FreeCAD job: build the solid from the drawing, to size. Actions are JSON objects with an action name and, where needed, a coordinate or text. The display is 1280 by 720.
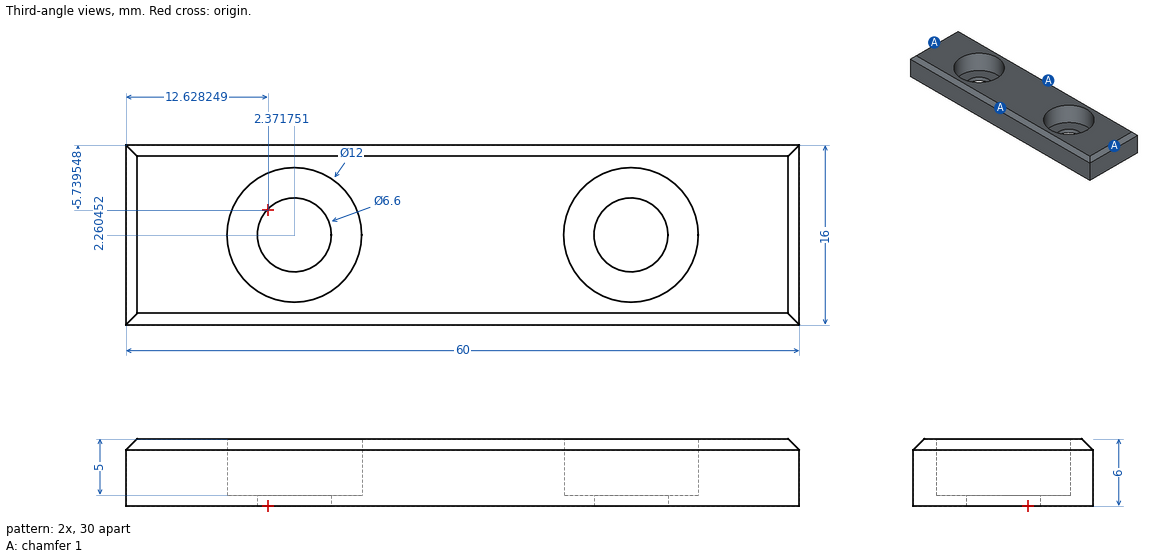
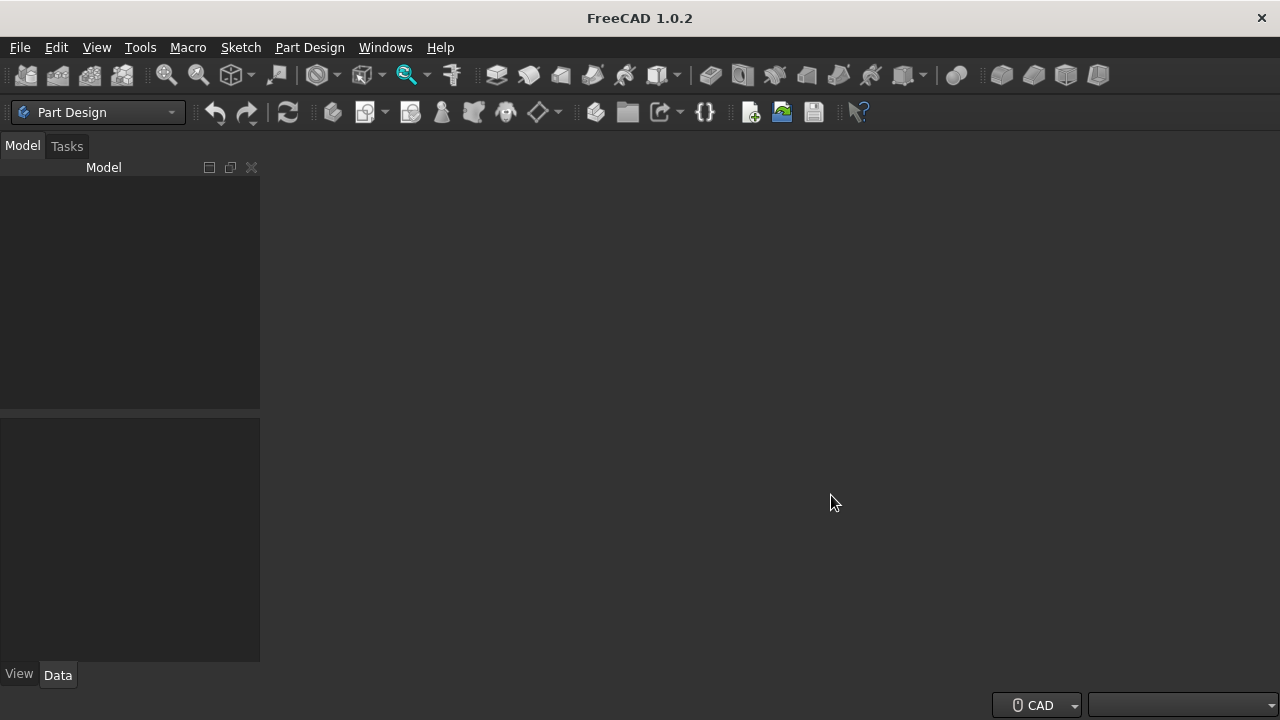
{"action": "left_click", "coordinate": [750, 112]}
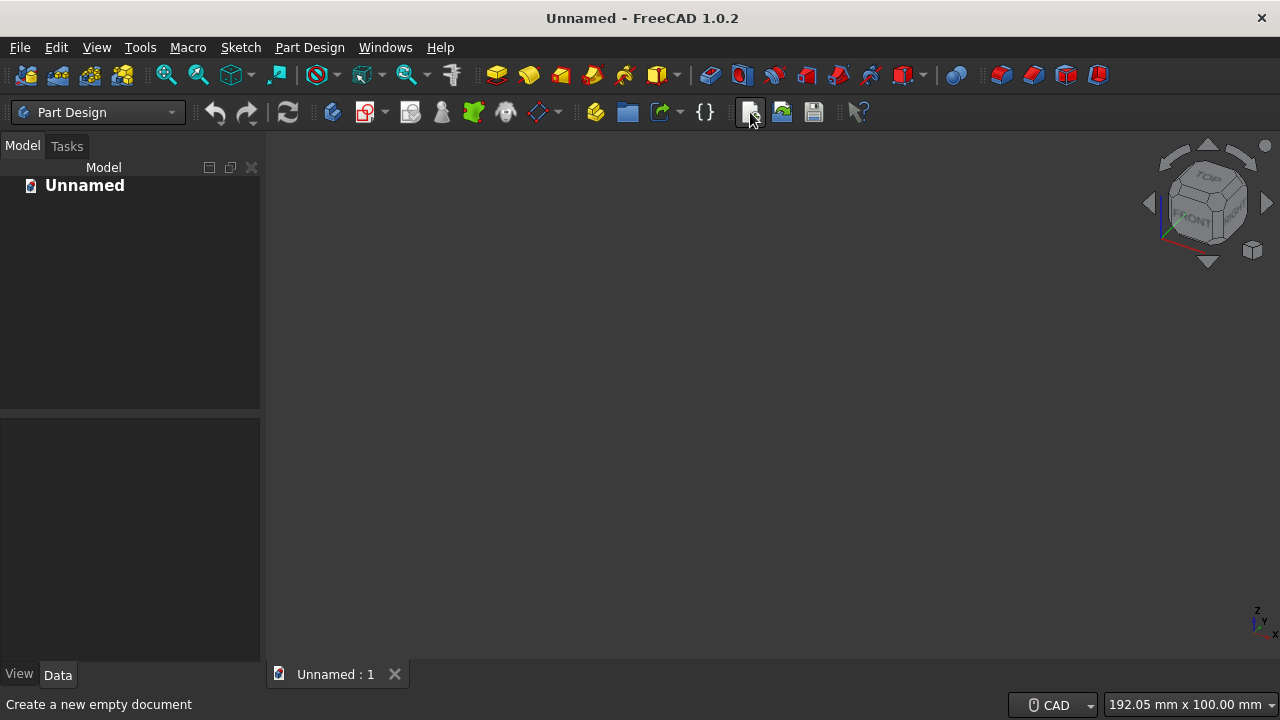
{"action": "left_click", "coordinate": [366, 112]}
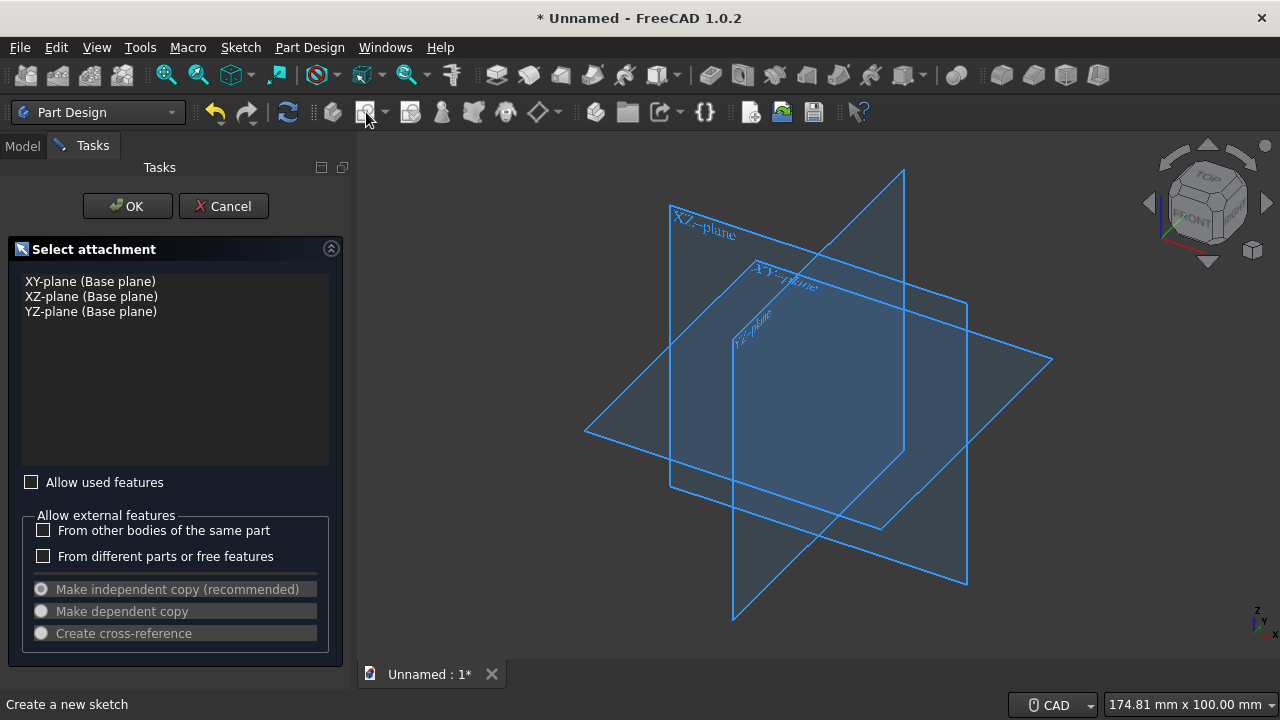
{"action": "left_click", "coordinate": [82, 282]}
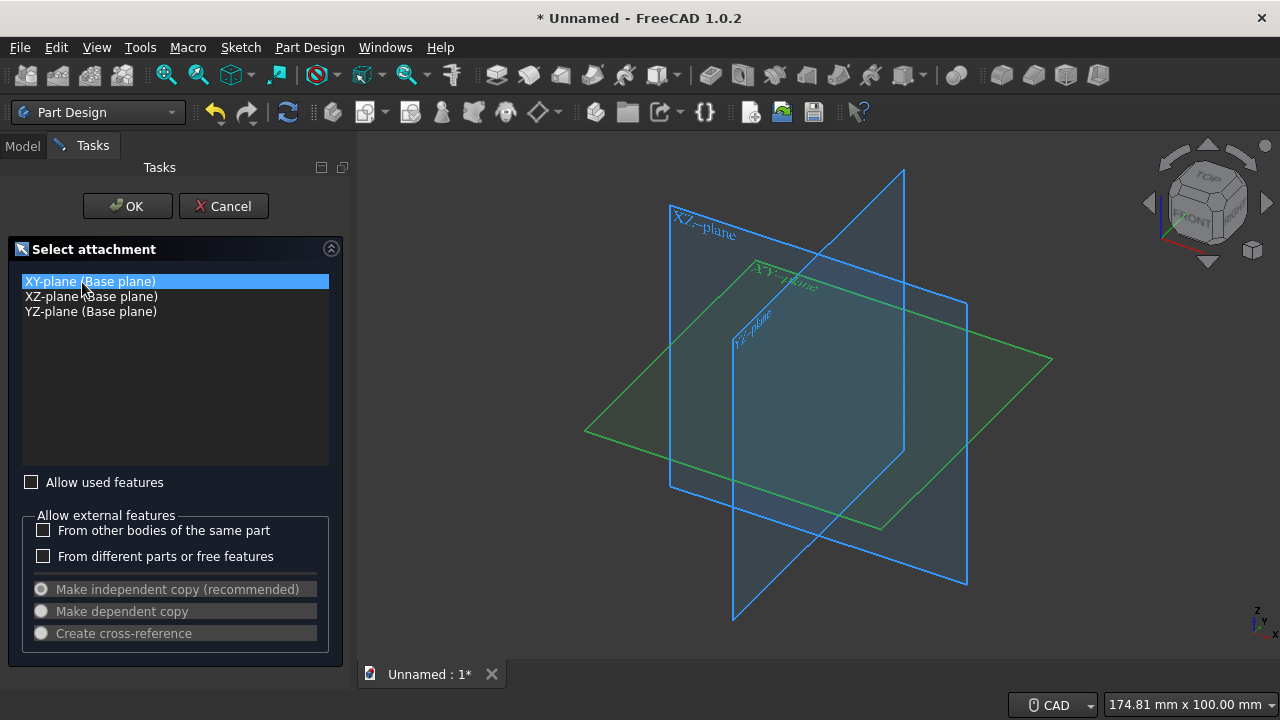
{"action": "left_click", "coordinate": [128, 206]}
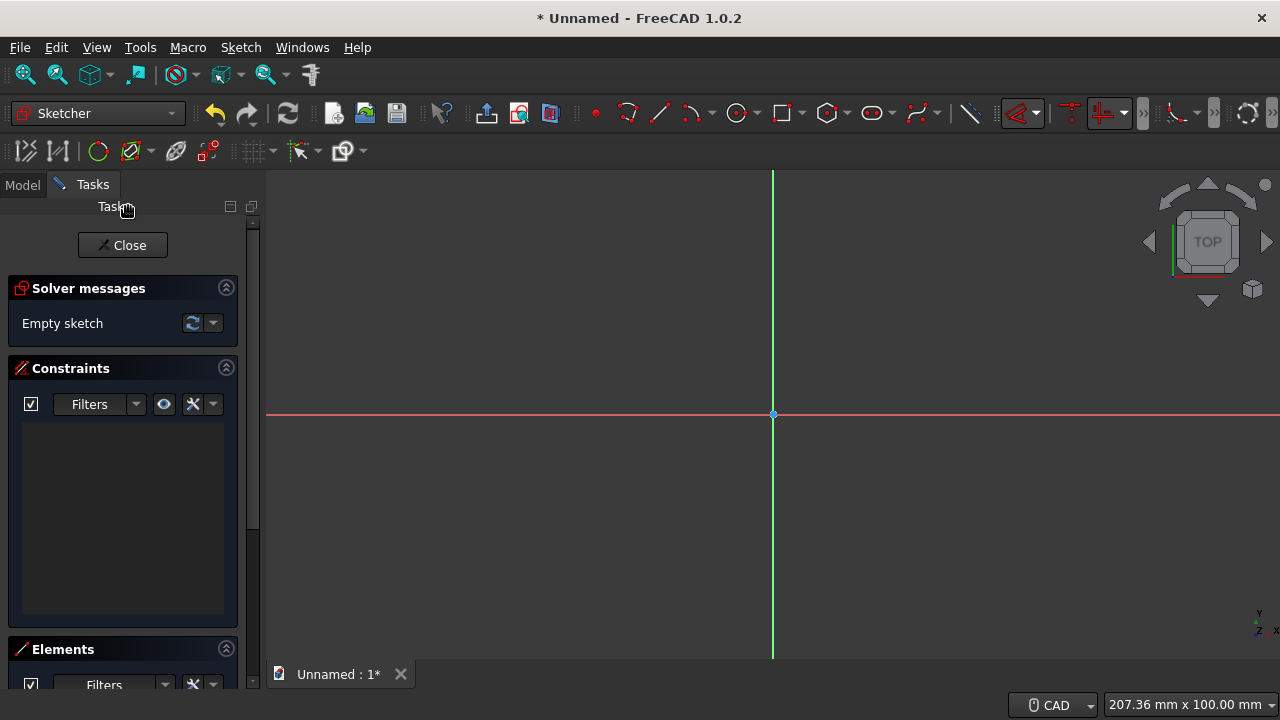
{"action": "scroll", "coordinate": [1045, 439], "scroll_direction": "up", "scroll_amount": 3}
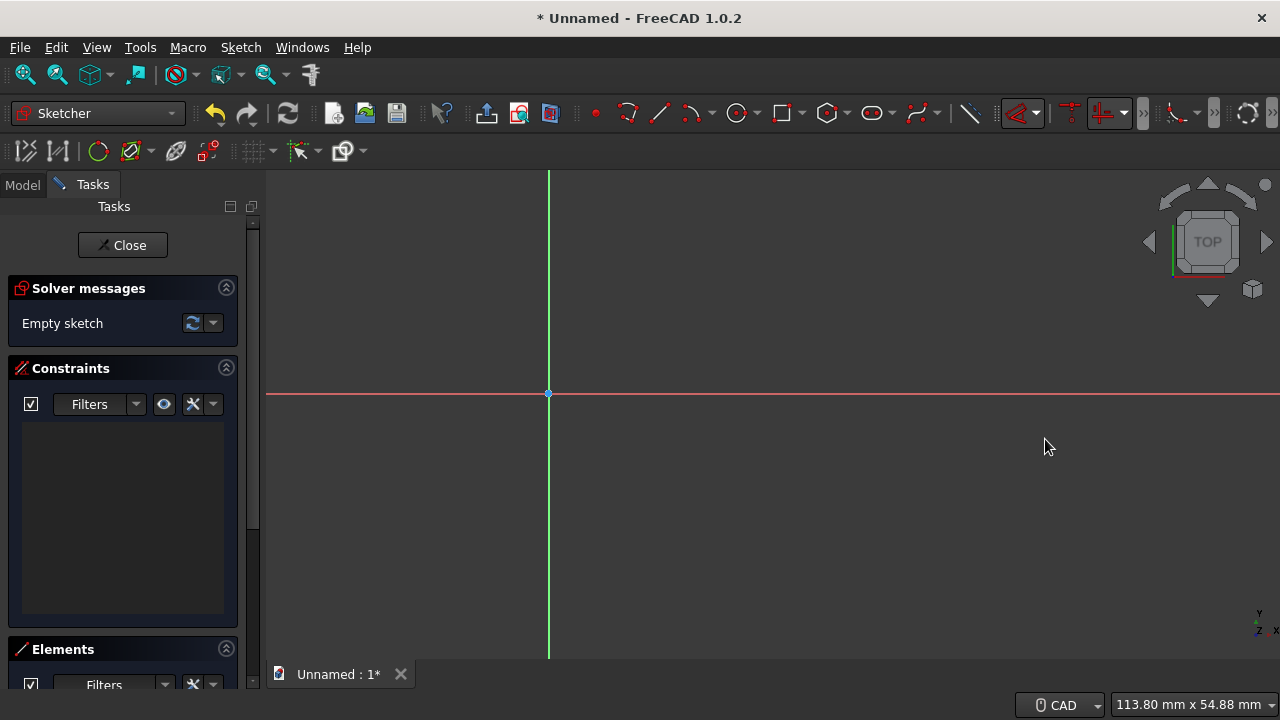
{"action": "left_click", "coordinate": [782, 114]}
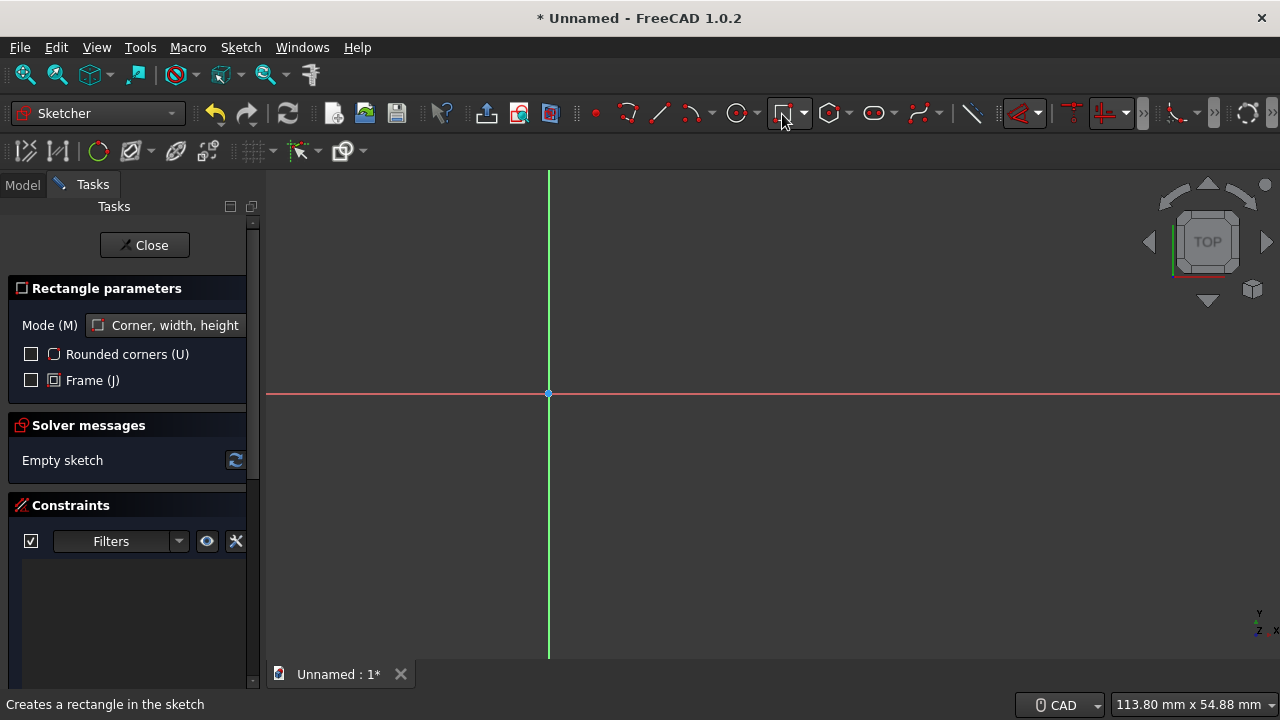
{"action": "left_click", "coordinate": [436, 343]}
{"action": "mouse_move", "coordinate": [971, 485]}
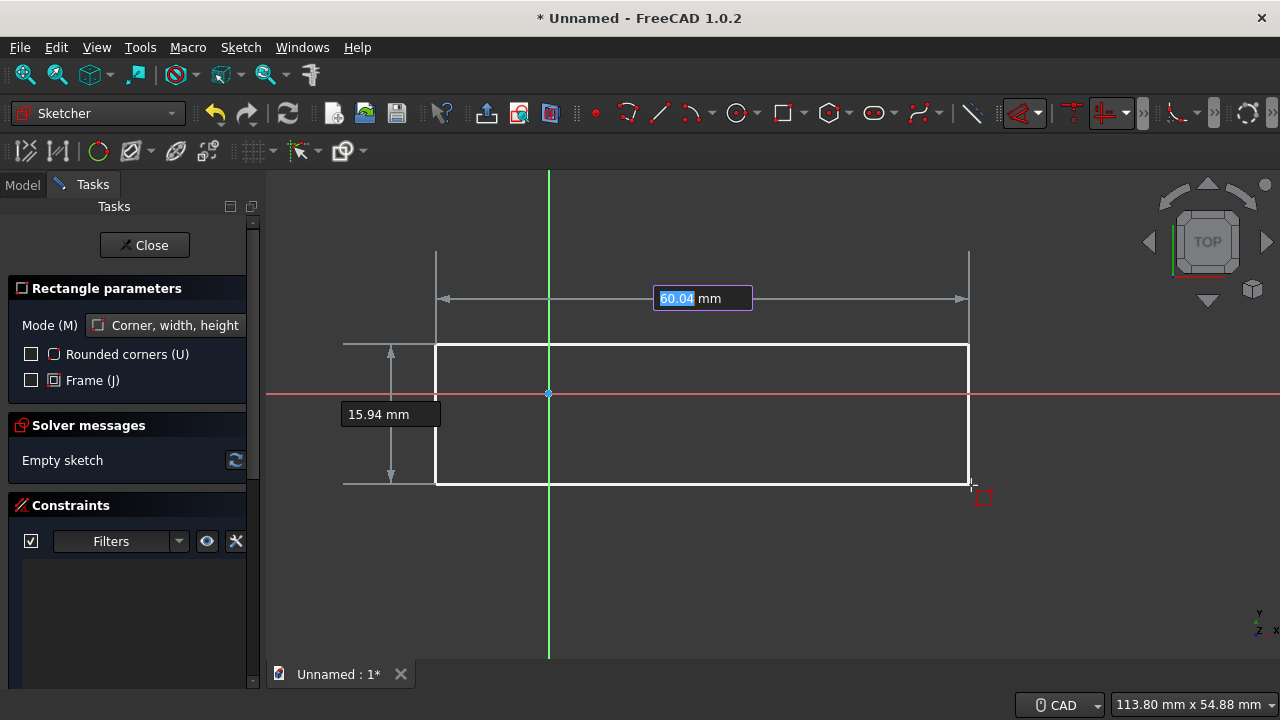
{"action": "type", "text": "60"}
{"action": "key", "text": "Tab"}
{"action": "type", "text": "16"}
{"action": "key", "text": "Return"}
{"action": "key", "text": "Escape"}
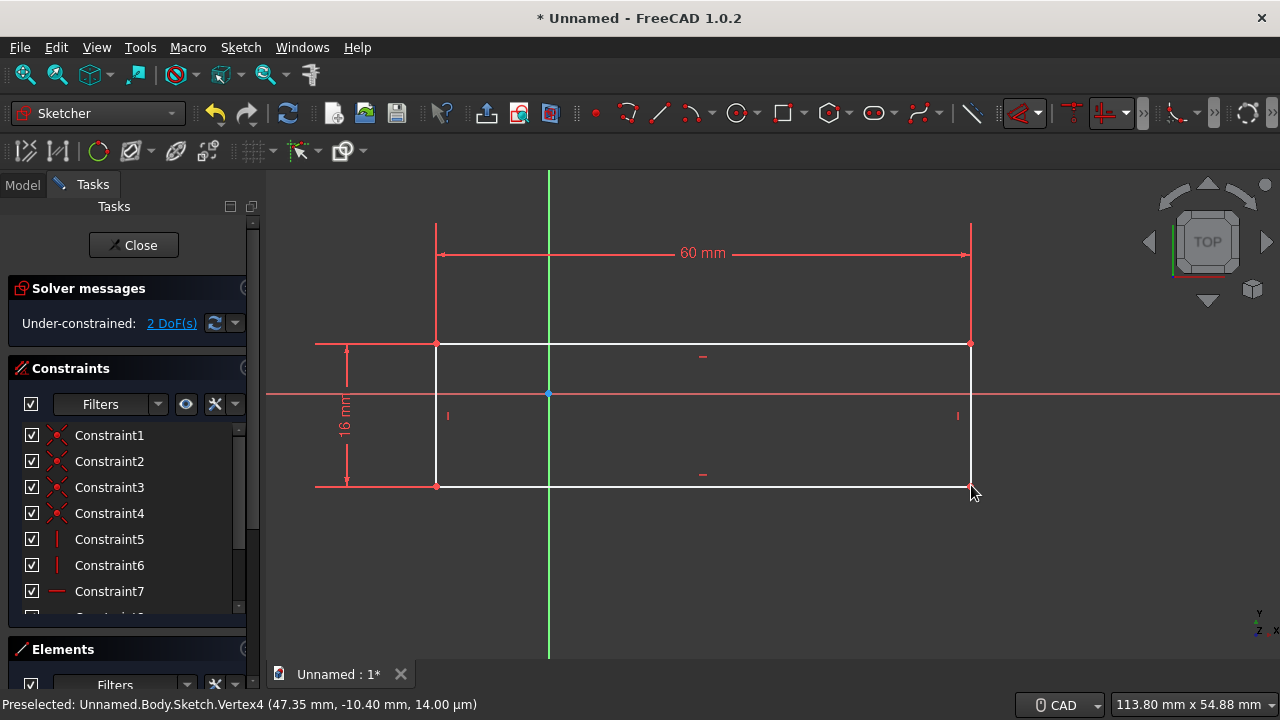
{"action": "left_click", "coordinate": [1018, 114]}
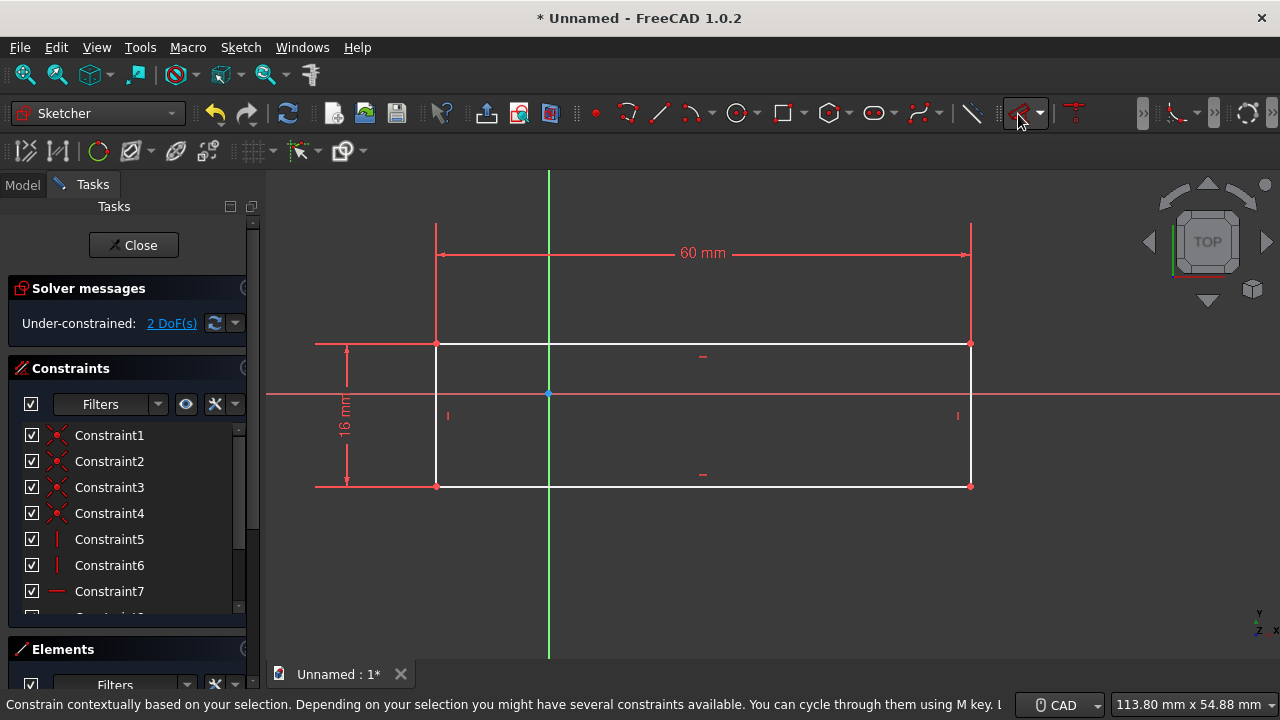
{"action": "left_click", "coordinate": [436, 344]}
{"action": "left_click", "coordinate": [402, 369]}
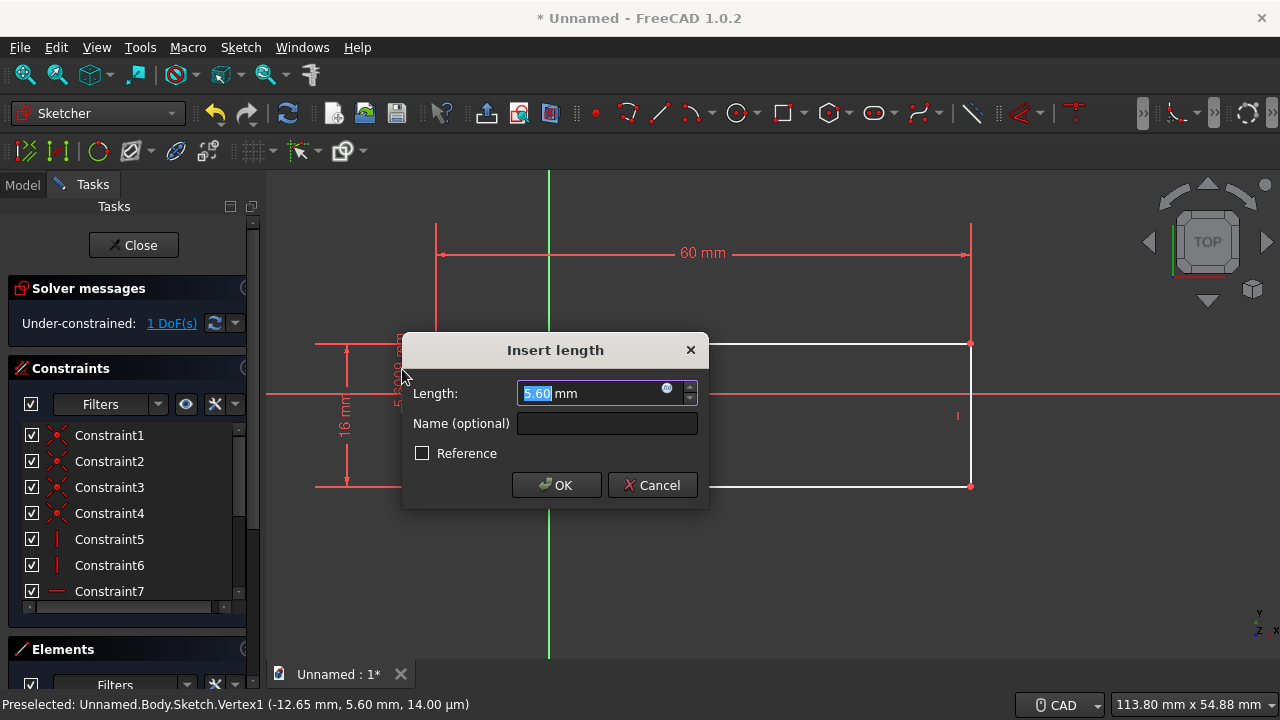
{"action": "type", "text": "5.739548"}
{"action": "key", "text": "Return"}